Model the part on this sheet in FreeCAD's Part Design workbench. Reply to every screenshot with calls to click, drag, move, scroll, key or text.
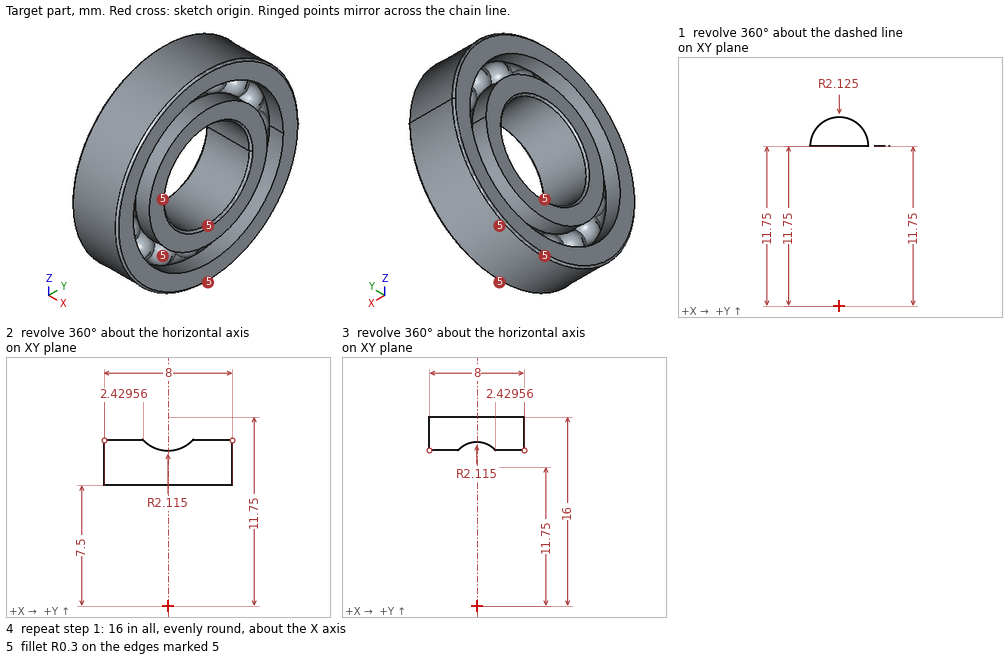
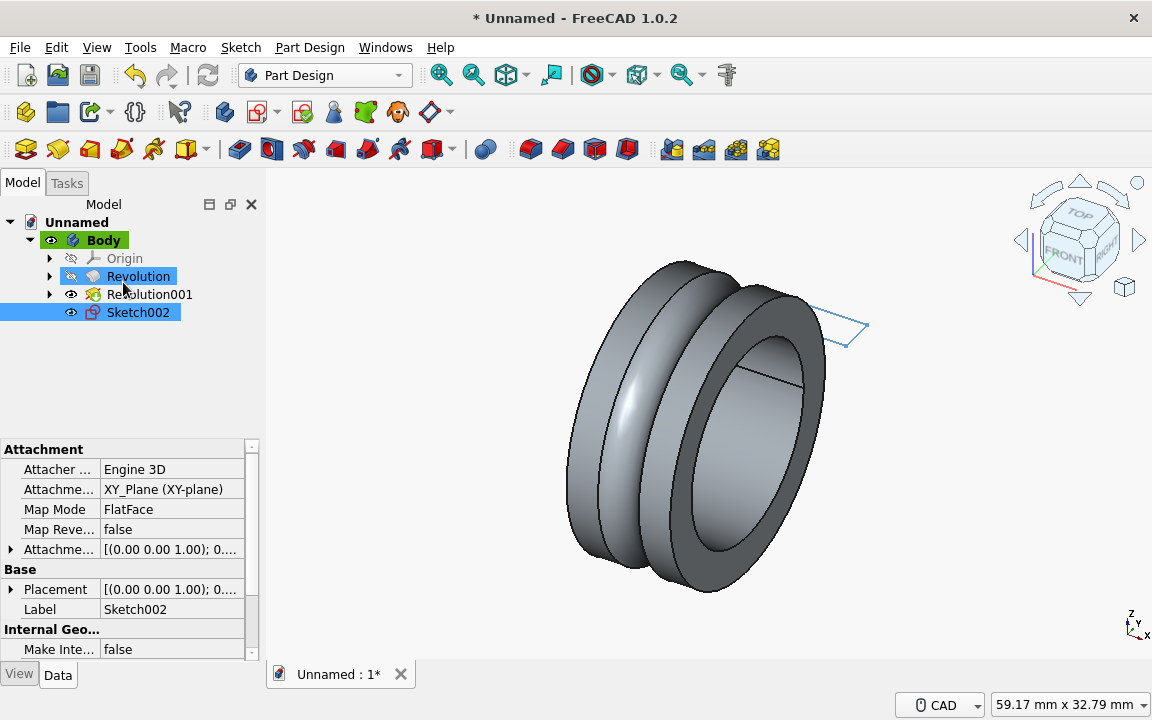
click(58, 150)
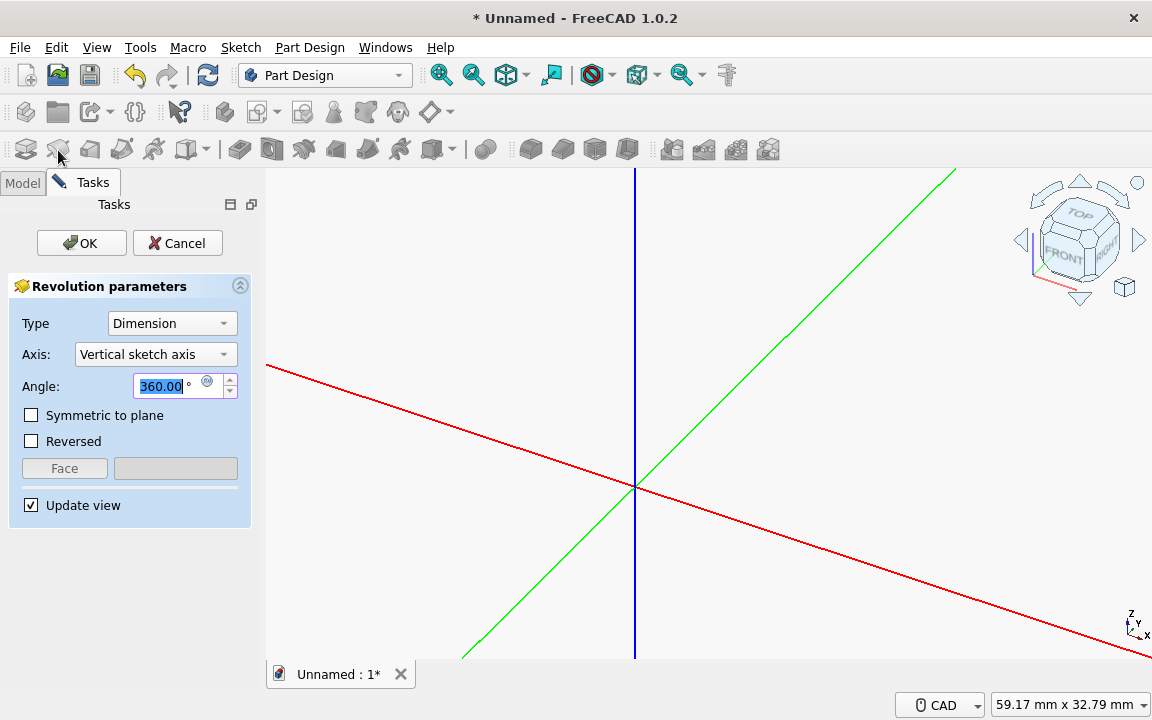
click(156, 354)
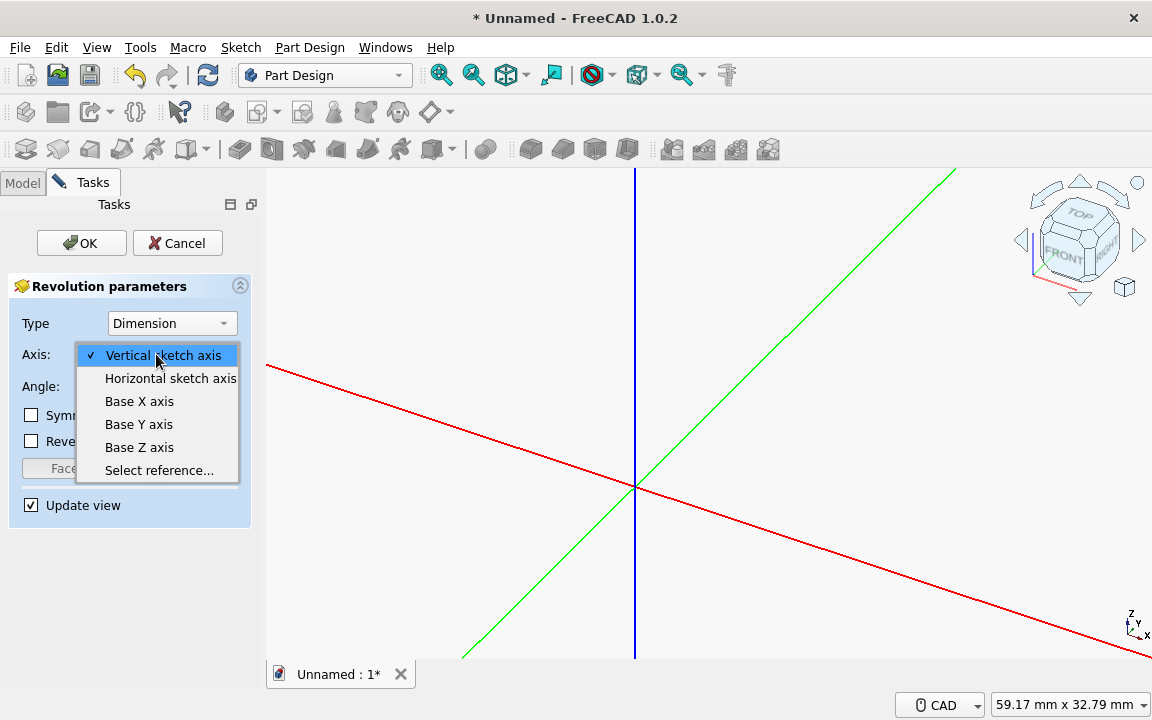
click(156, 378)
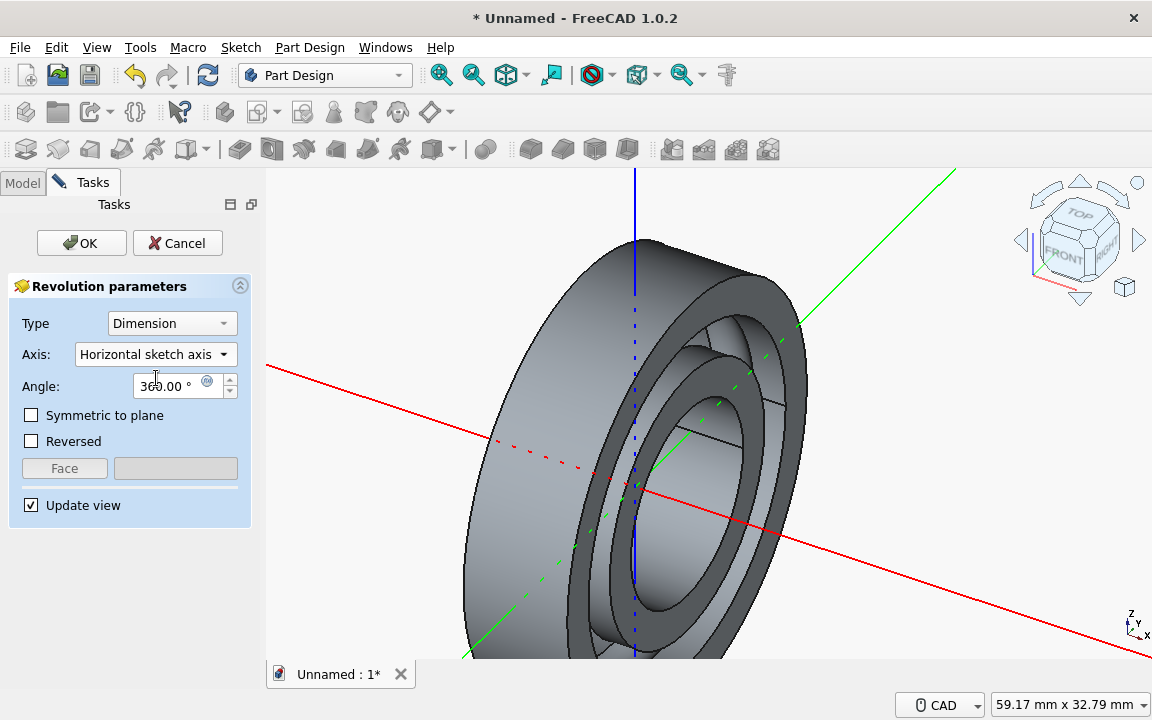
click(82, 243)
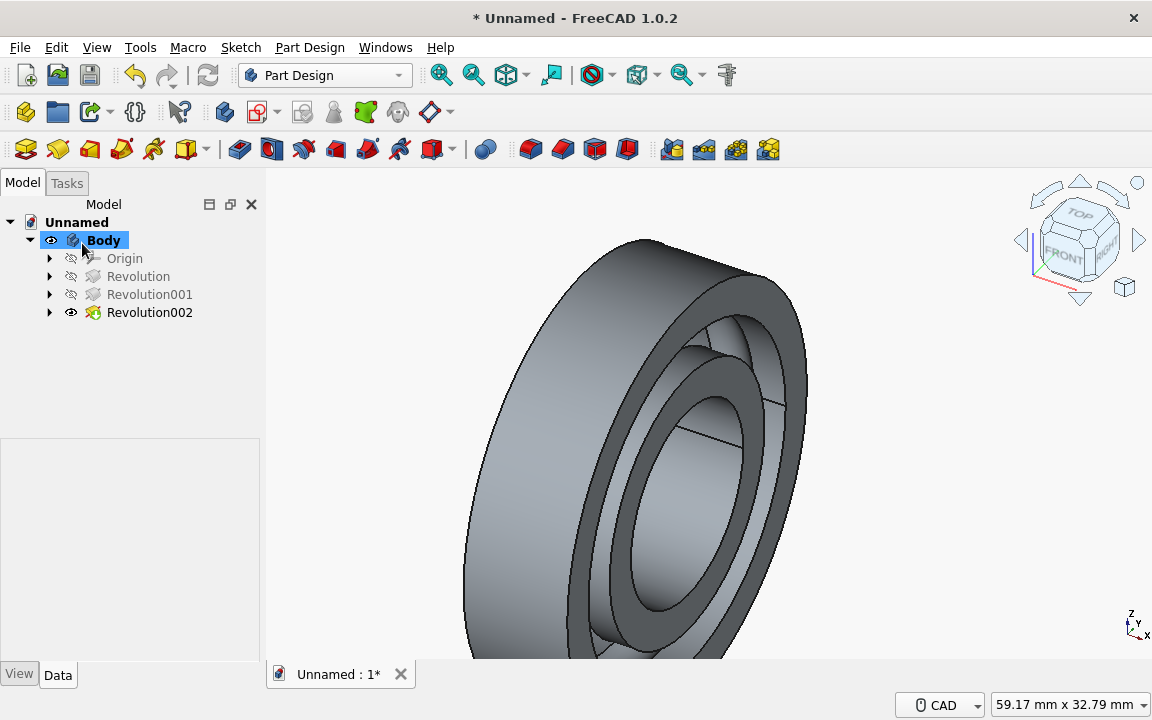
click(442, 76)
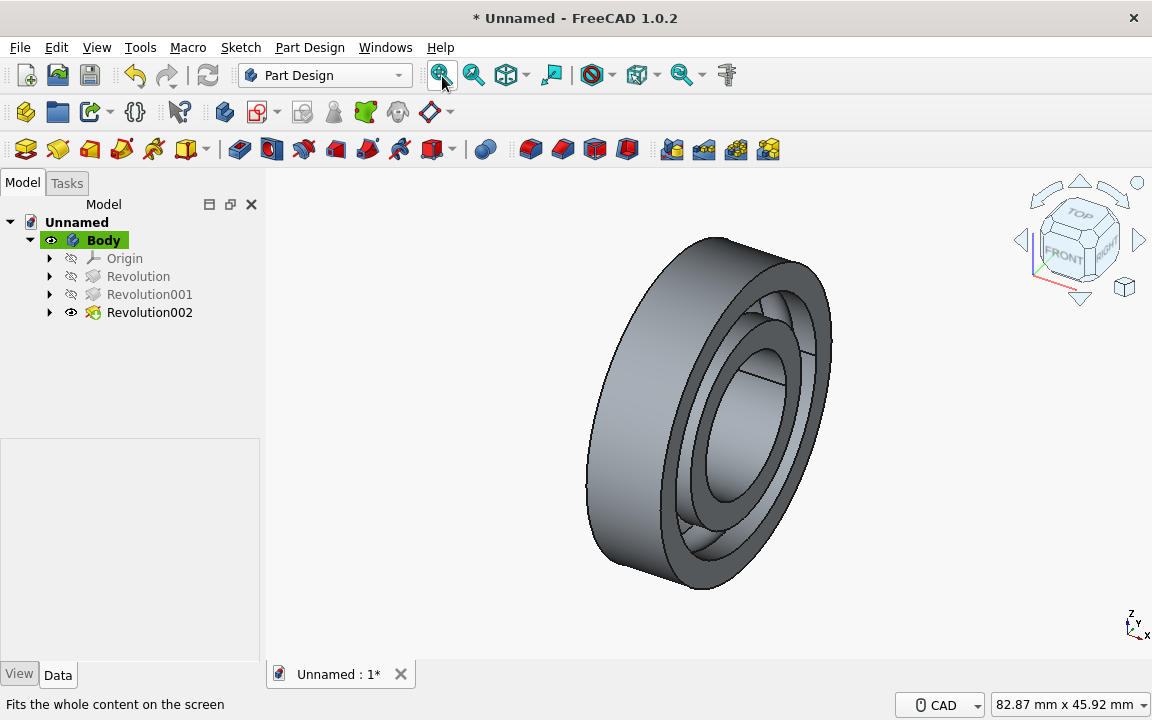
click(116, 276)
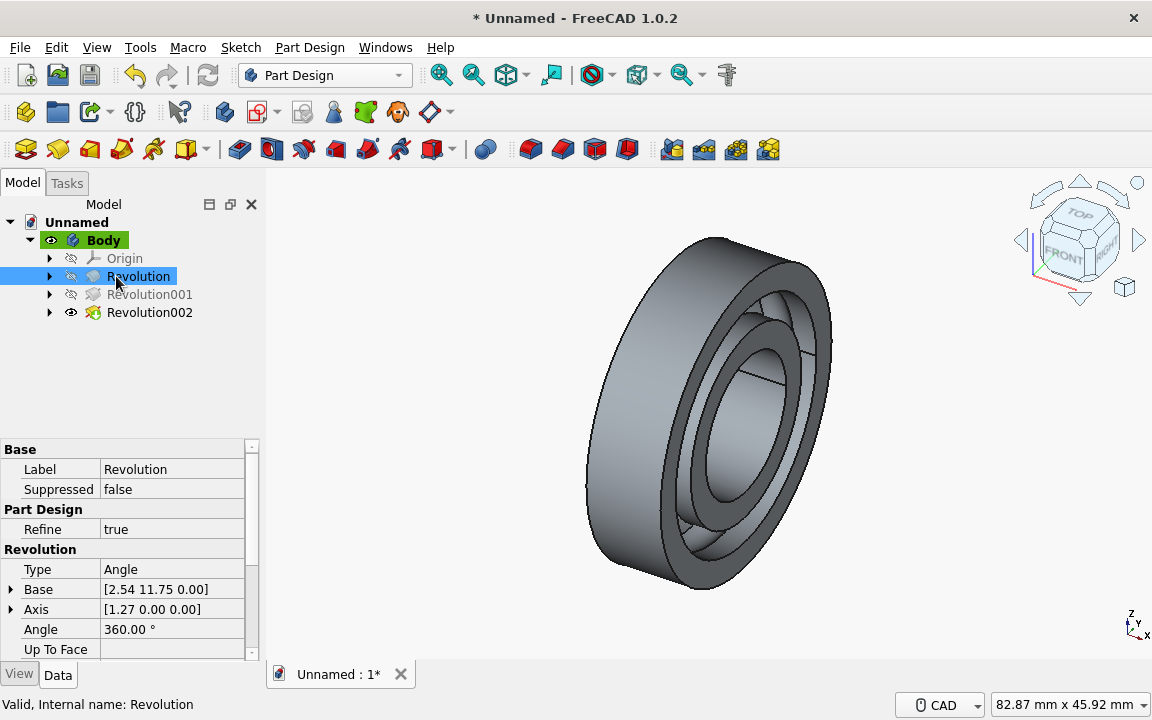
click(736, 150)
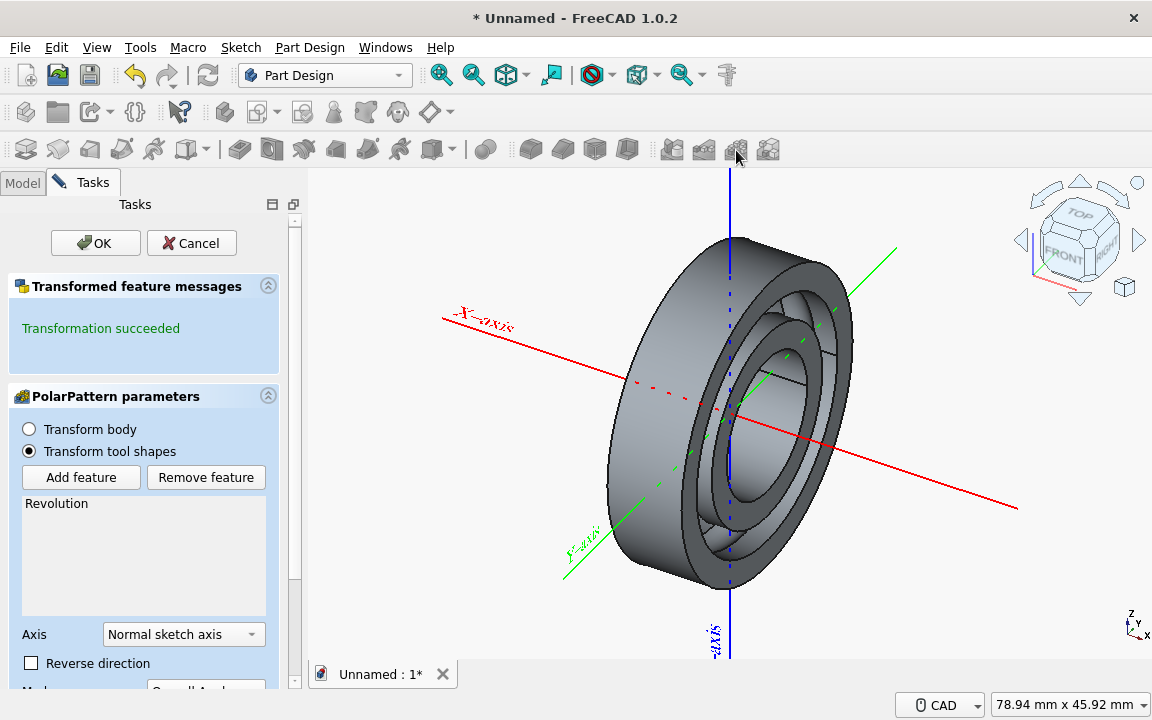
click(184, 634)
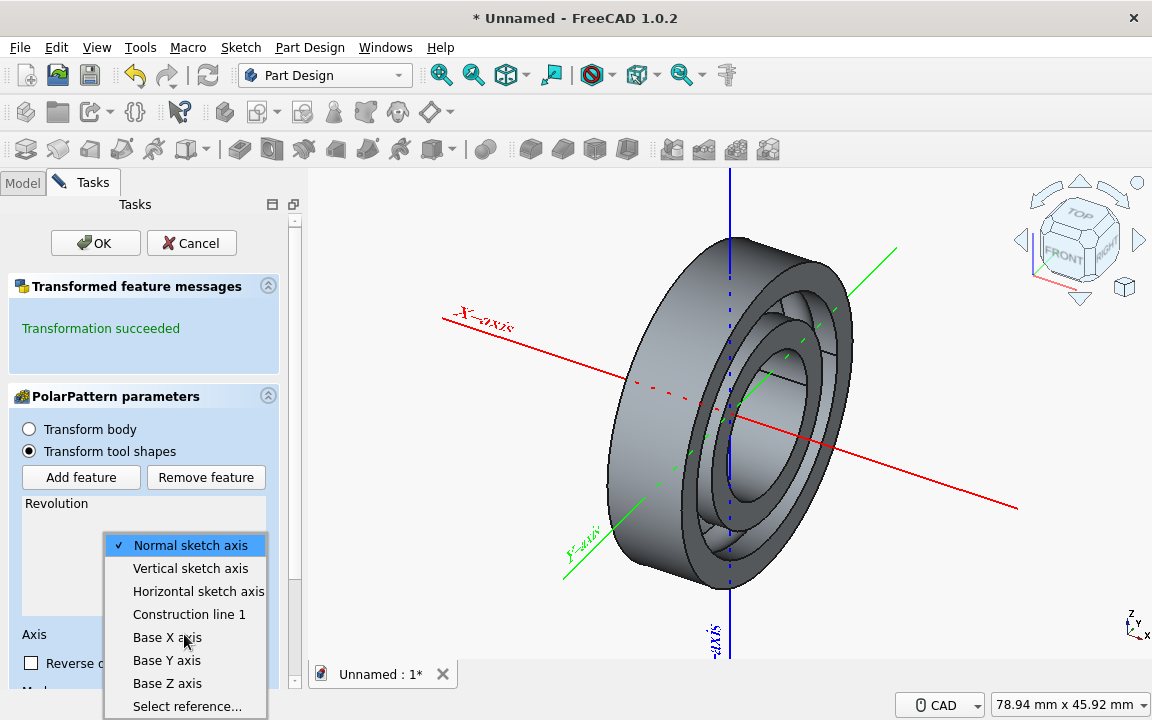
click(184, 638)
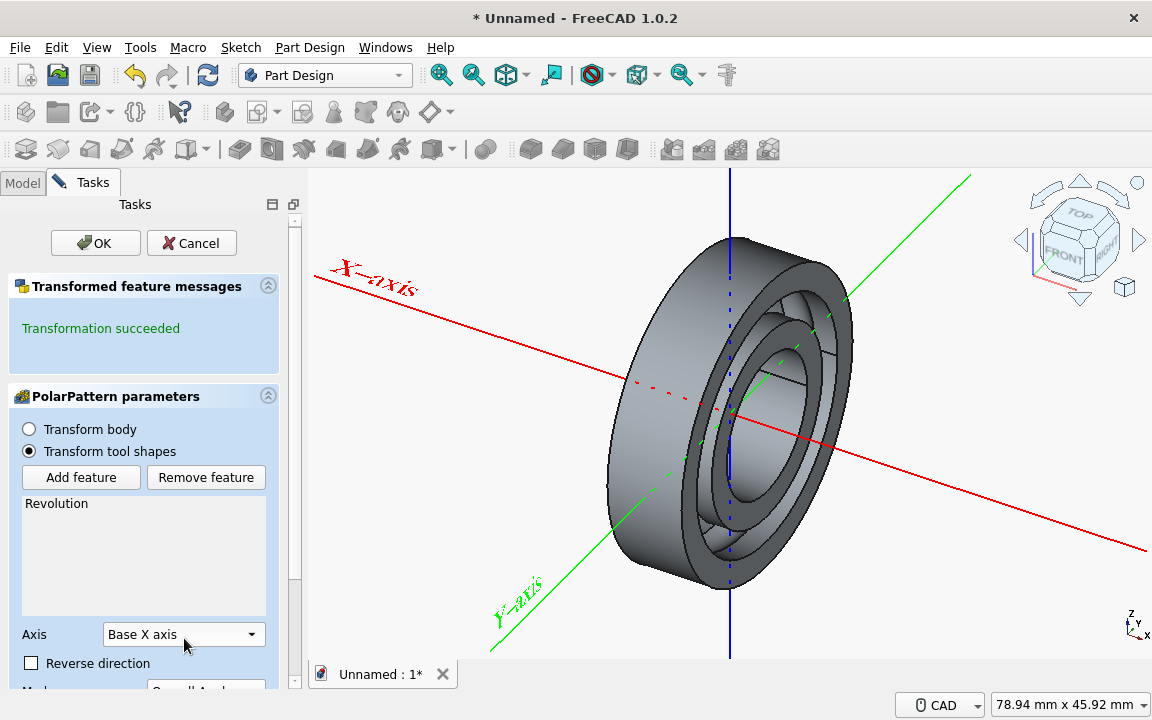
scroll(295, 451, down, 3)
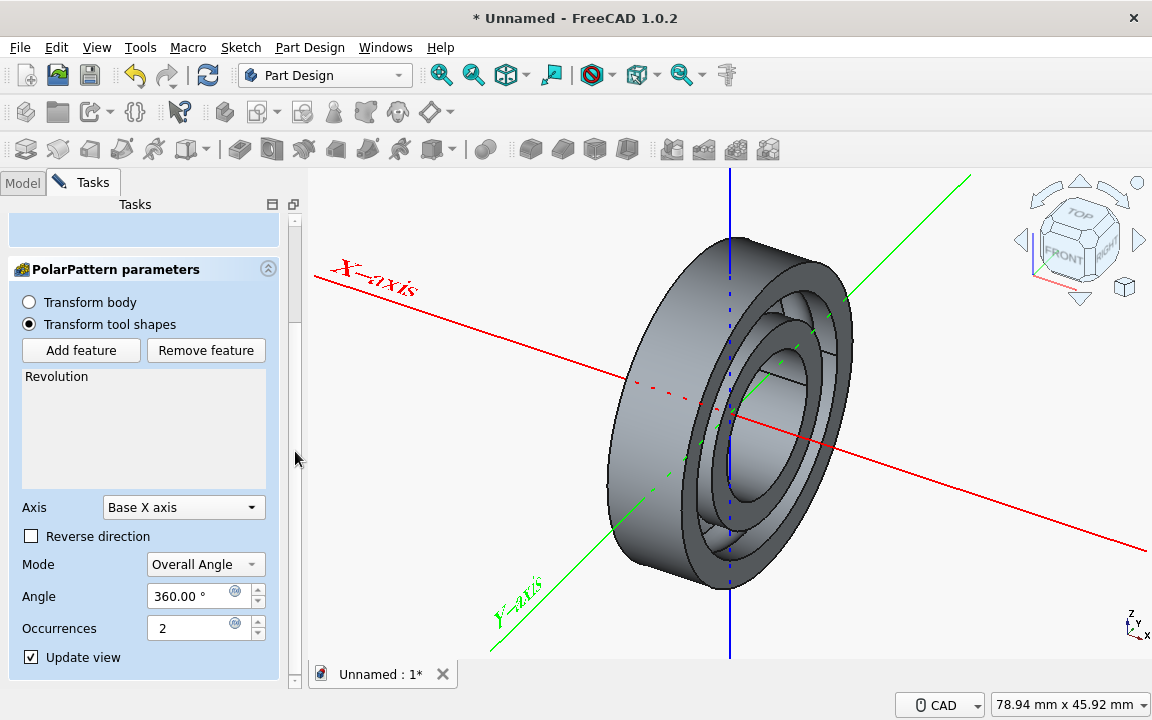
triple_click(198, 628)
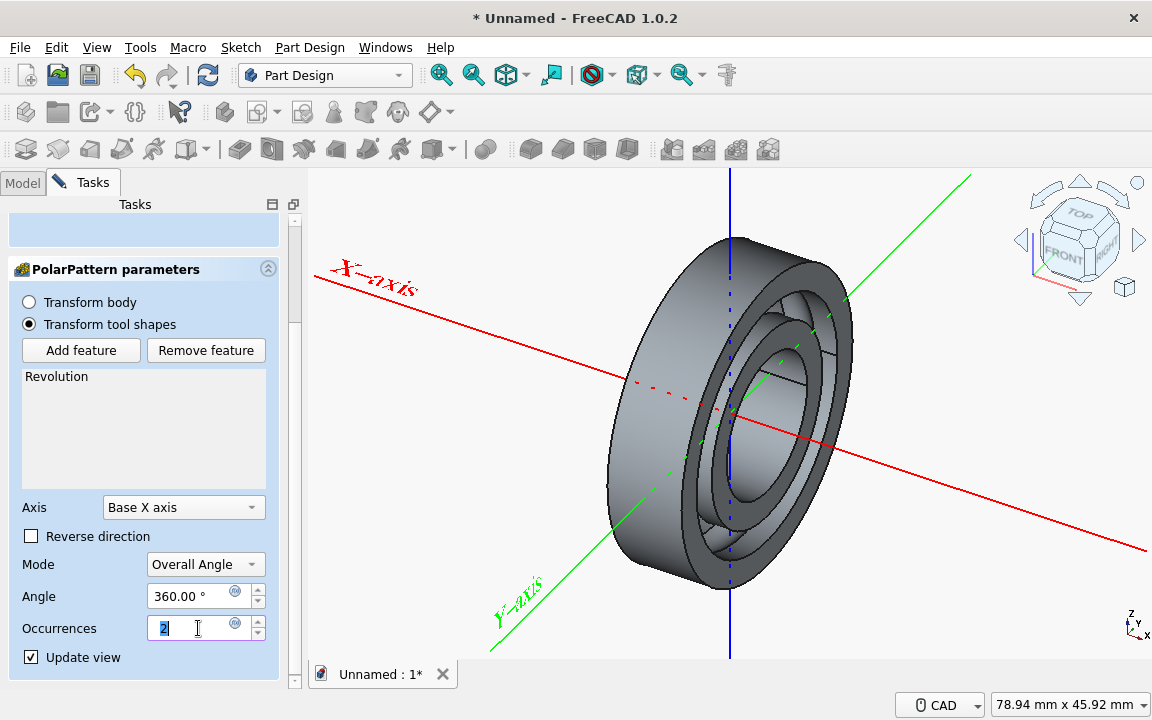
text(16)
key(Tab)